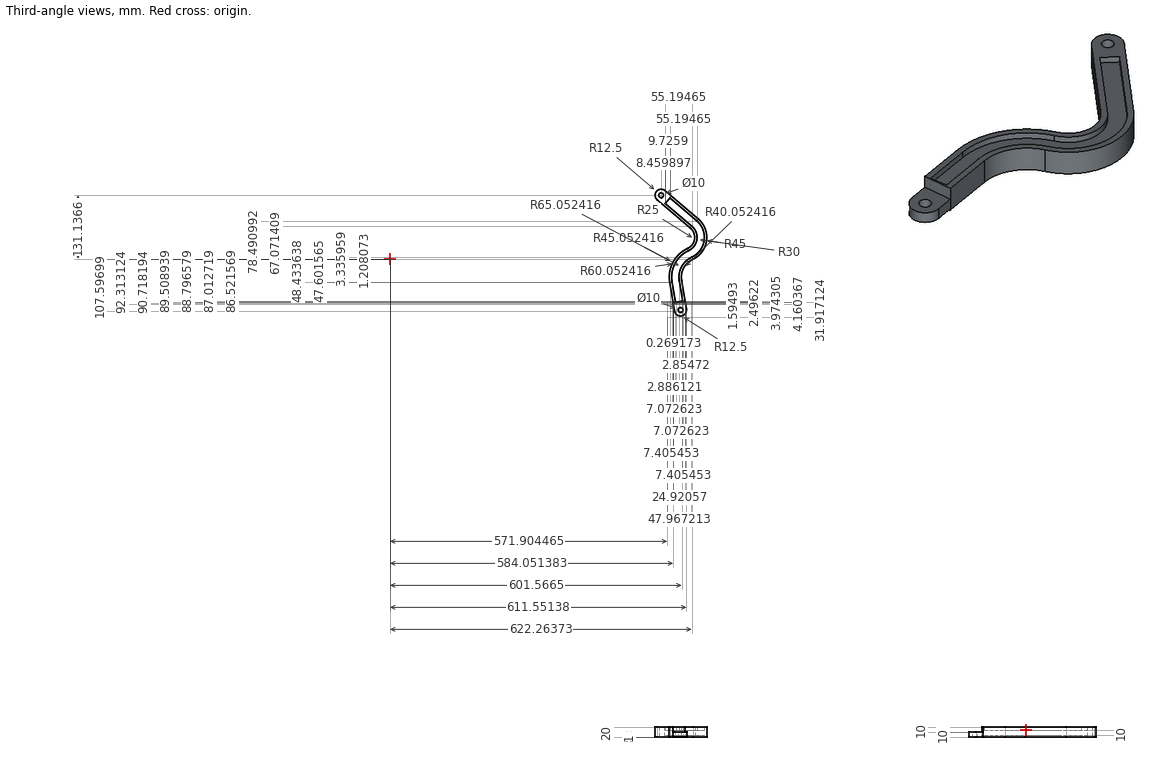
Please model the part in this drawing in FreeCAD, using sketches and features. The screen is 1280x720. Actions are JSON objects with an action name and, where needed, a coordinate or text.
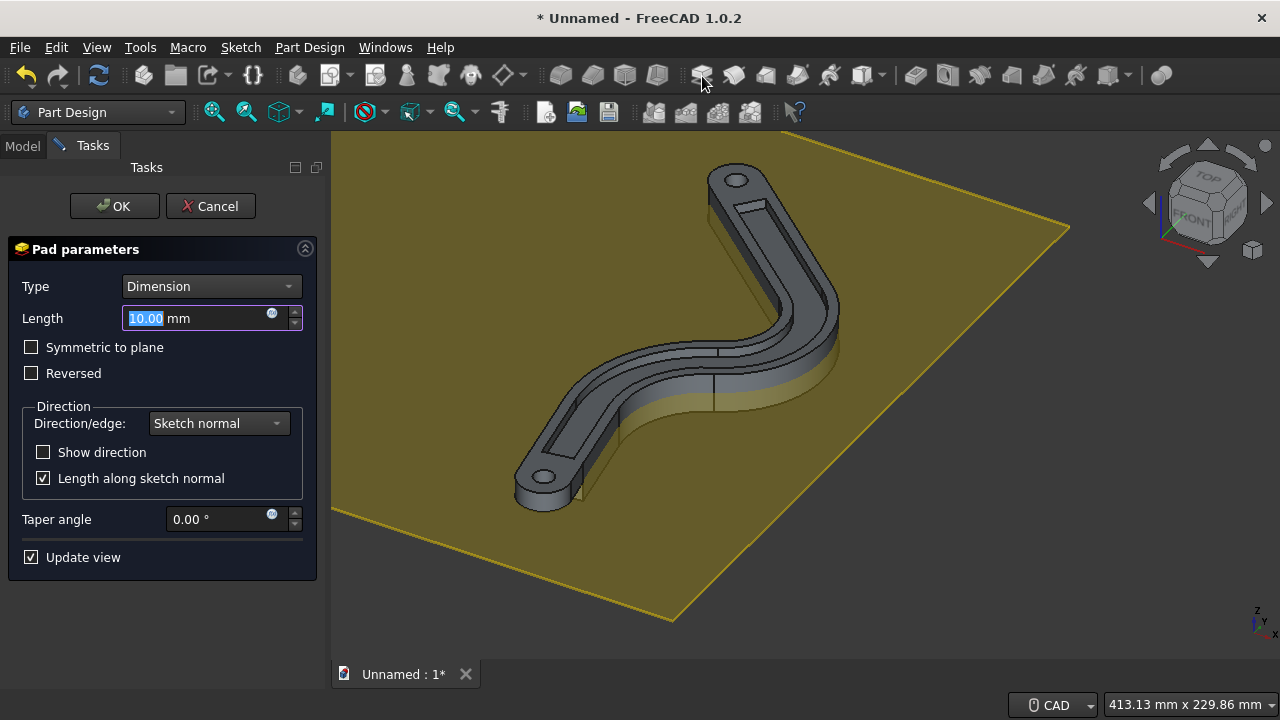
{"action": "type", "text": "10"}
{"action": "key", "text": "Tab"}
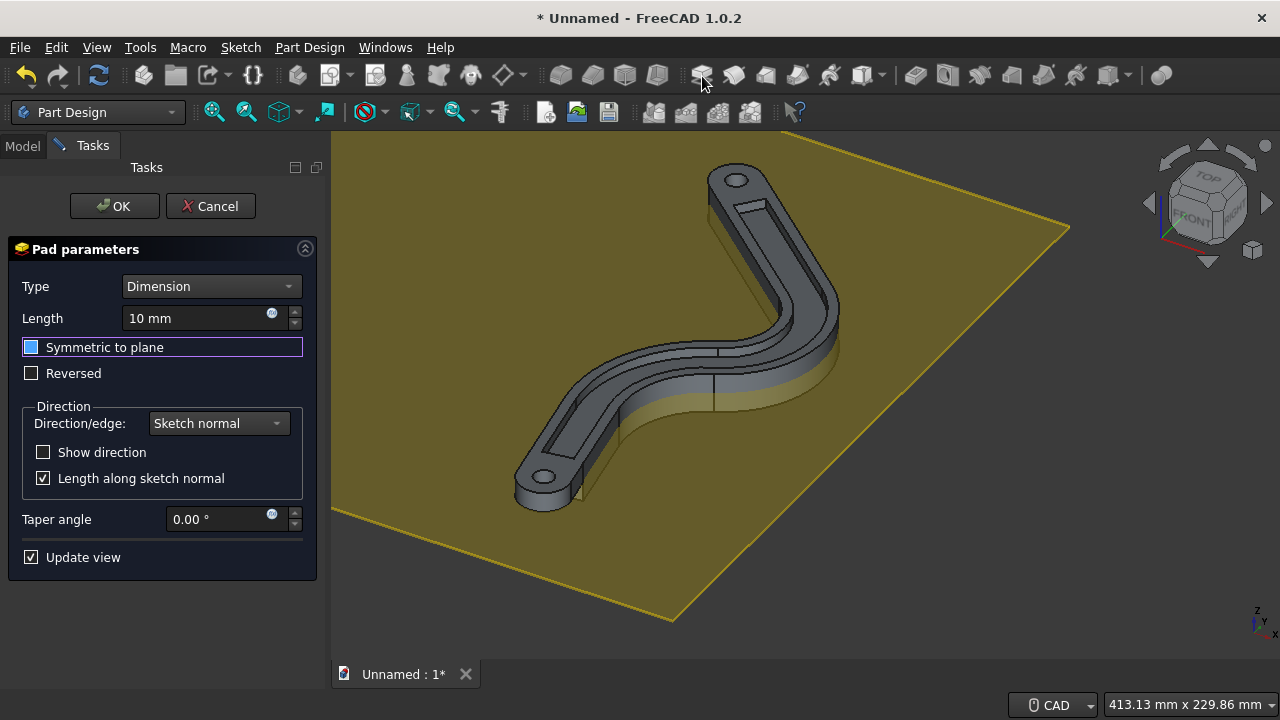
{"action": "left_click", "coordinate": [30, 373]}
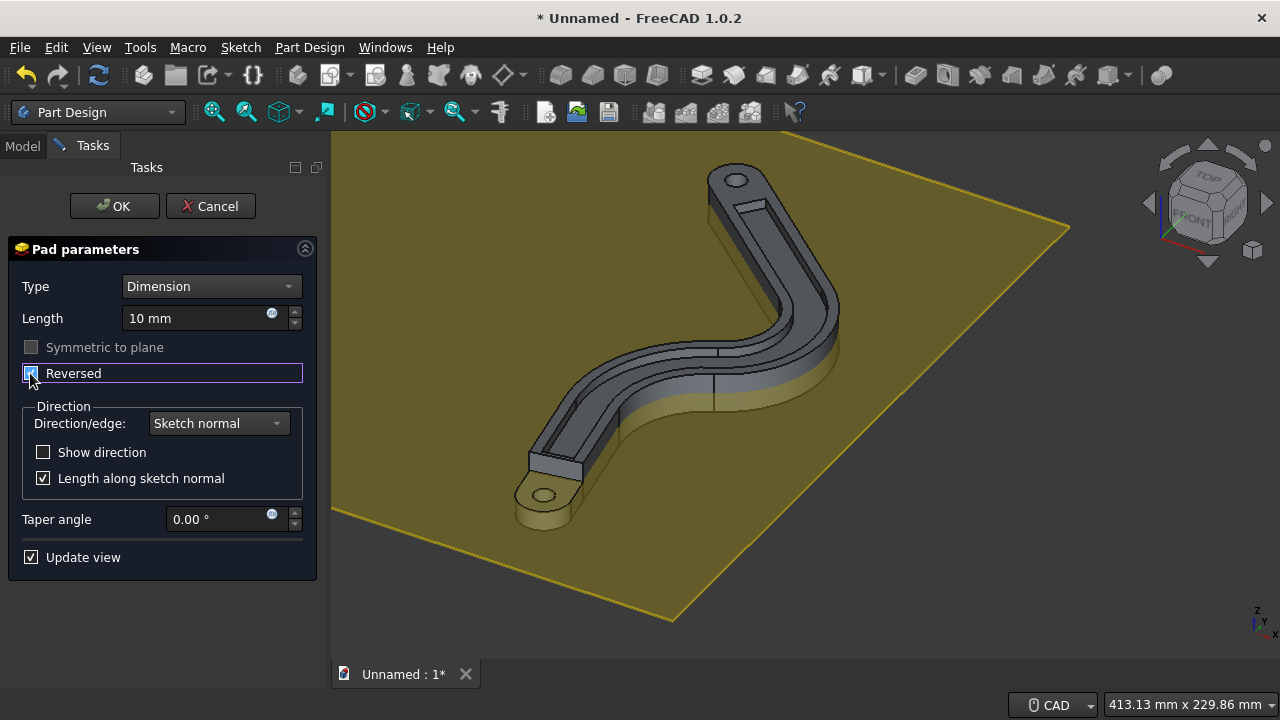
{"action": "left_click", "coordinate": [115, 206]}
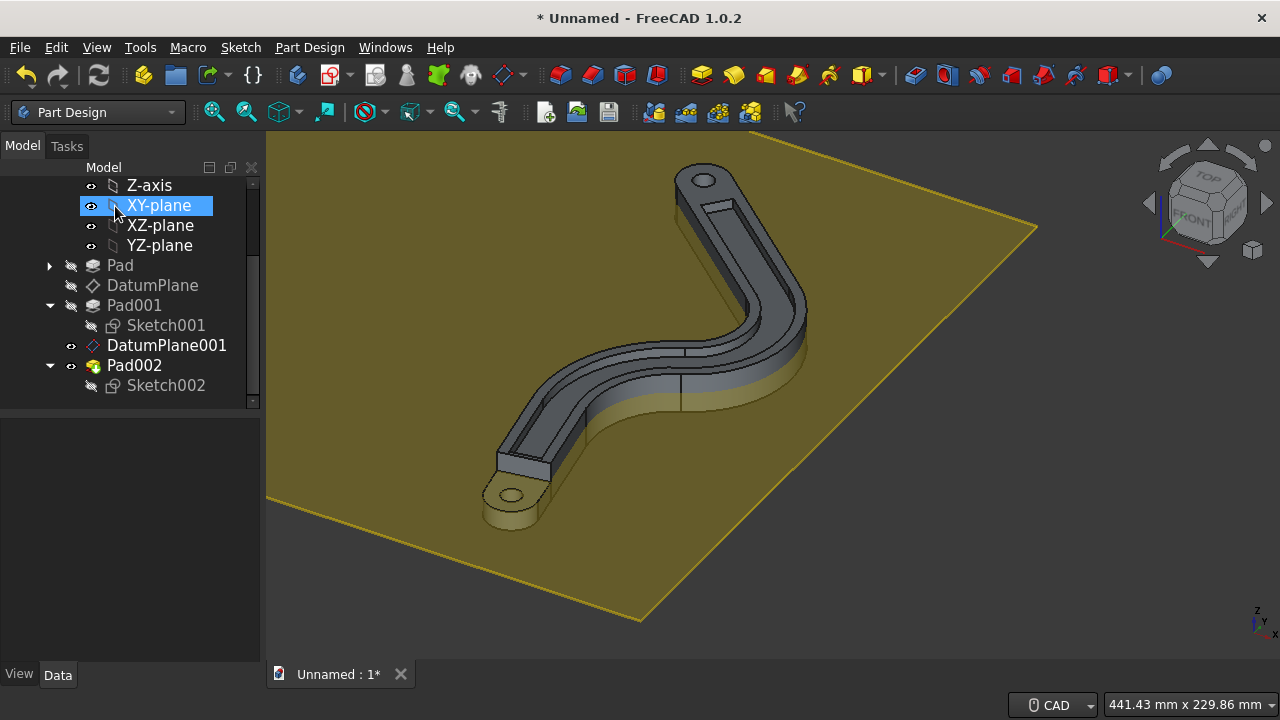
{"action": "left_click", "coordinate": [116, 346]}
{"action": "key", "text": "space"}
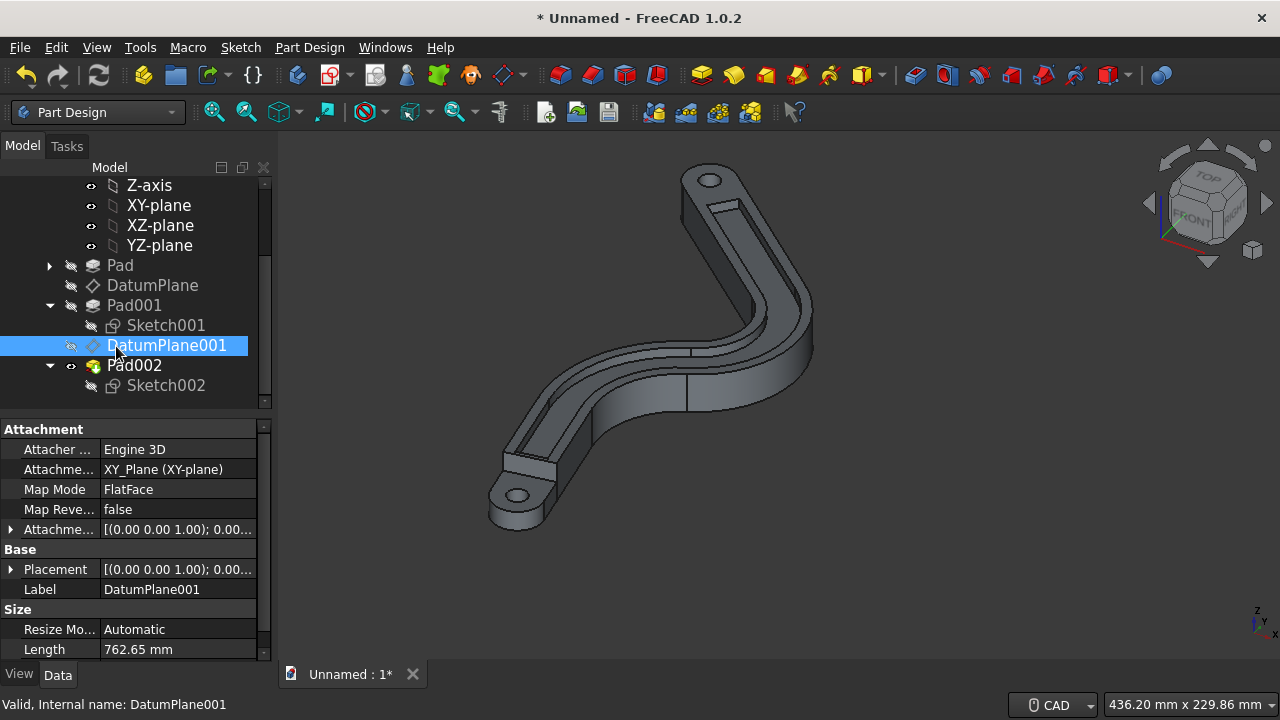
{"action": "key", "text": "5"}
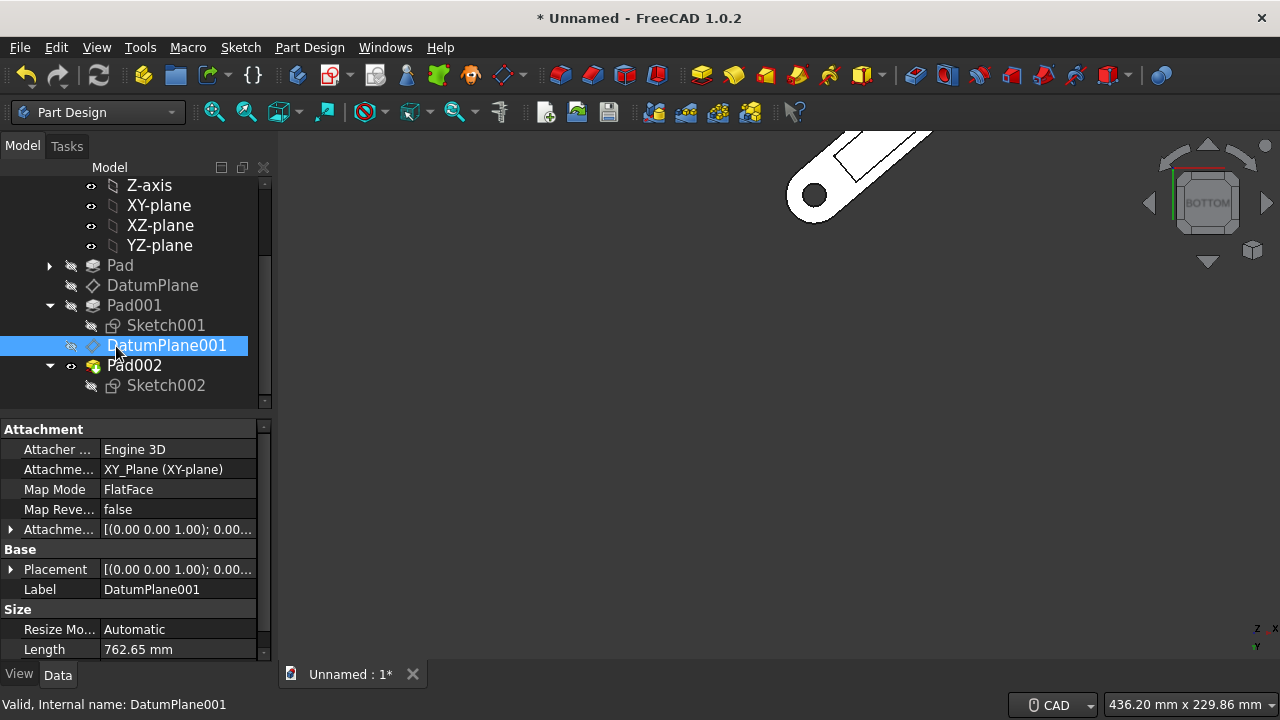
{"action": "left_click", "coordinate": [216, 112]}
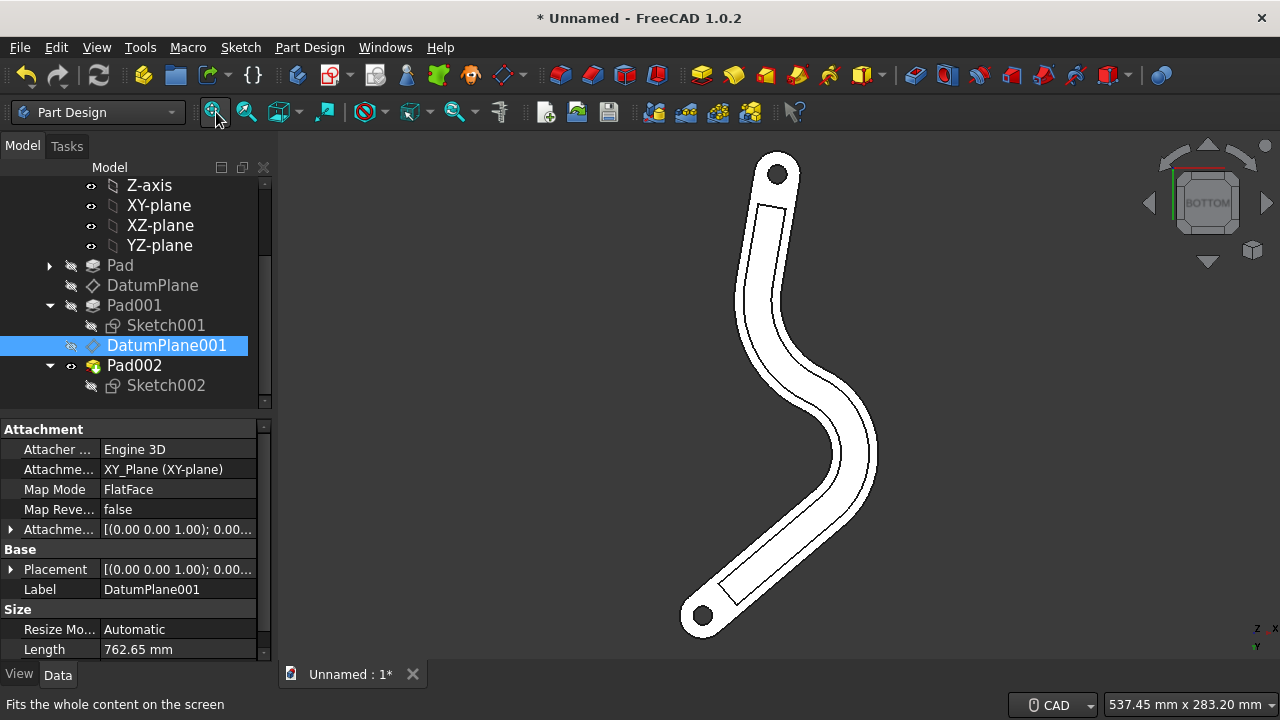
{"action": "left_click", "coordinate": [722, 603]}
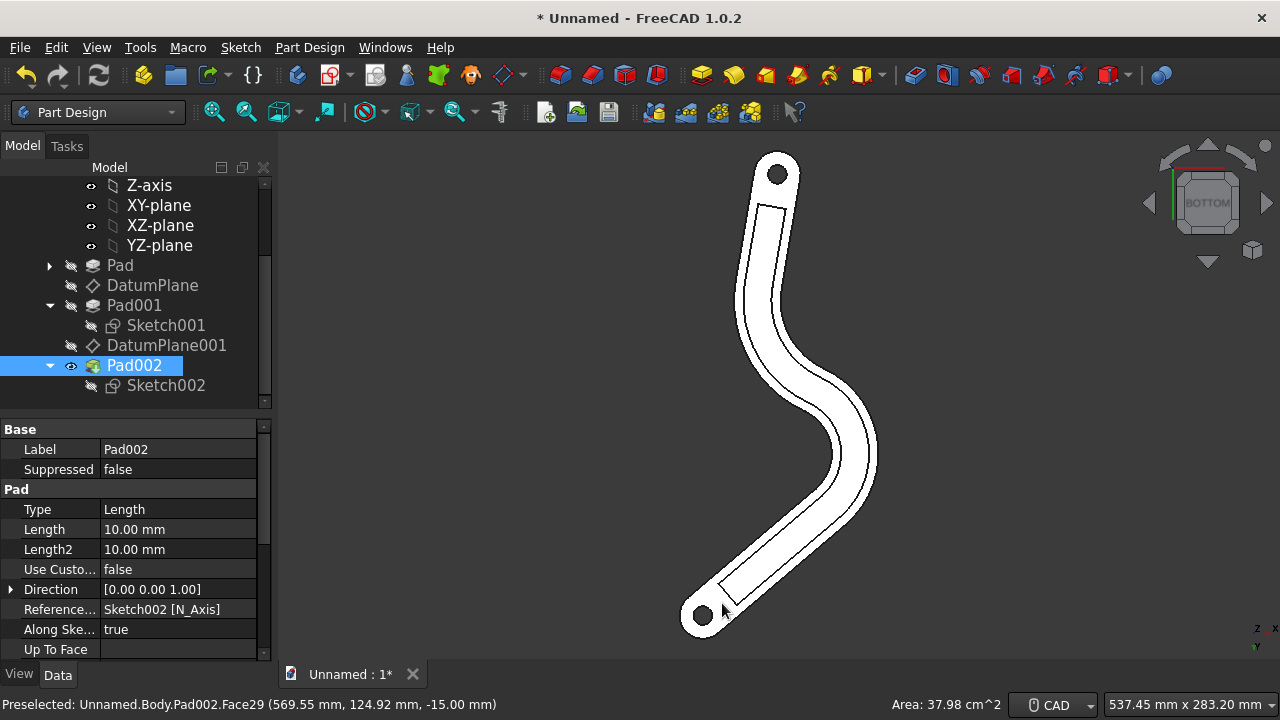
{"action": "left_click", "coordinate": [330, 76]}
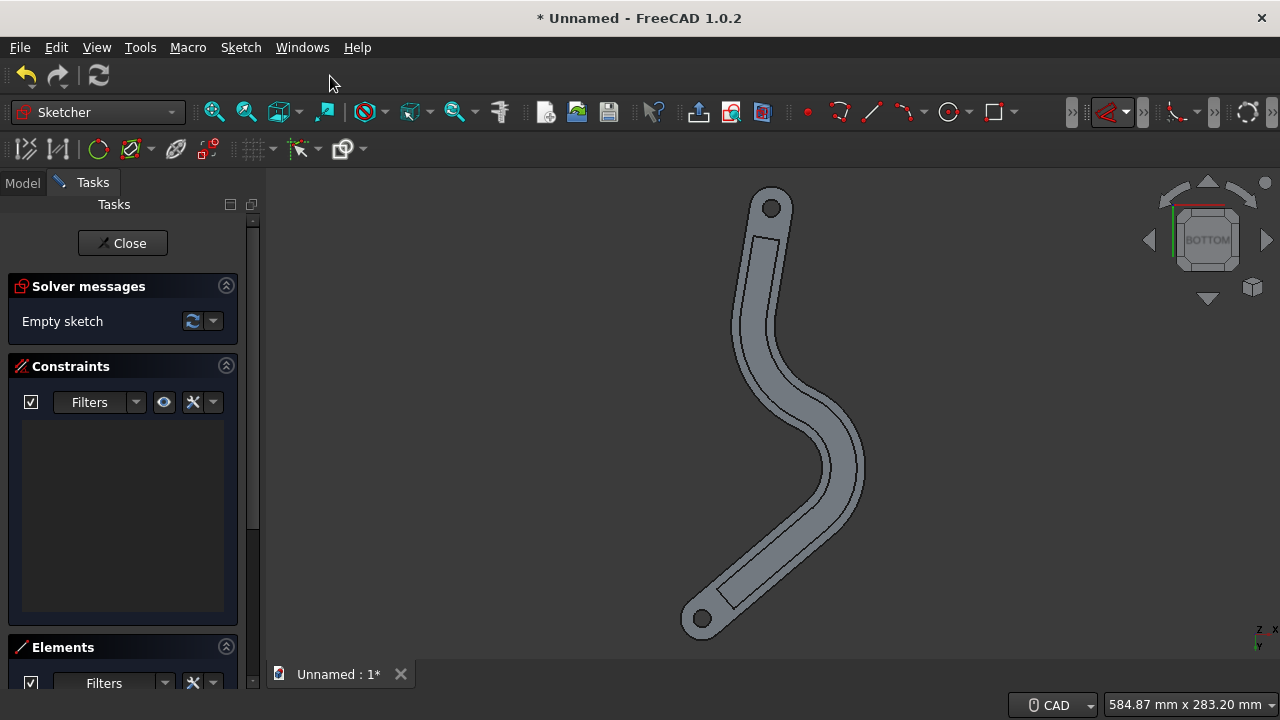
{"action": "scroll", "coordinate": [704, 414], "scroll_direction": "down", "scroll_amount": 5}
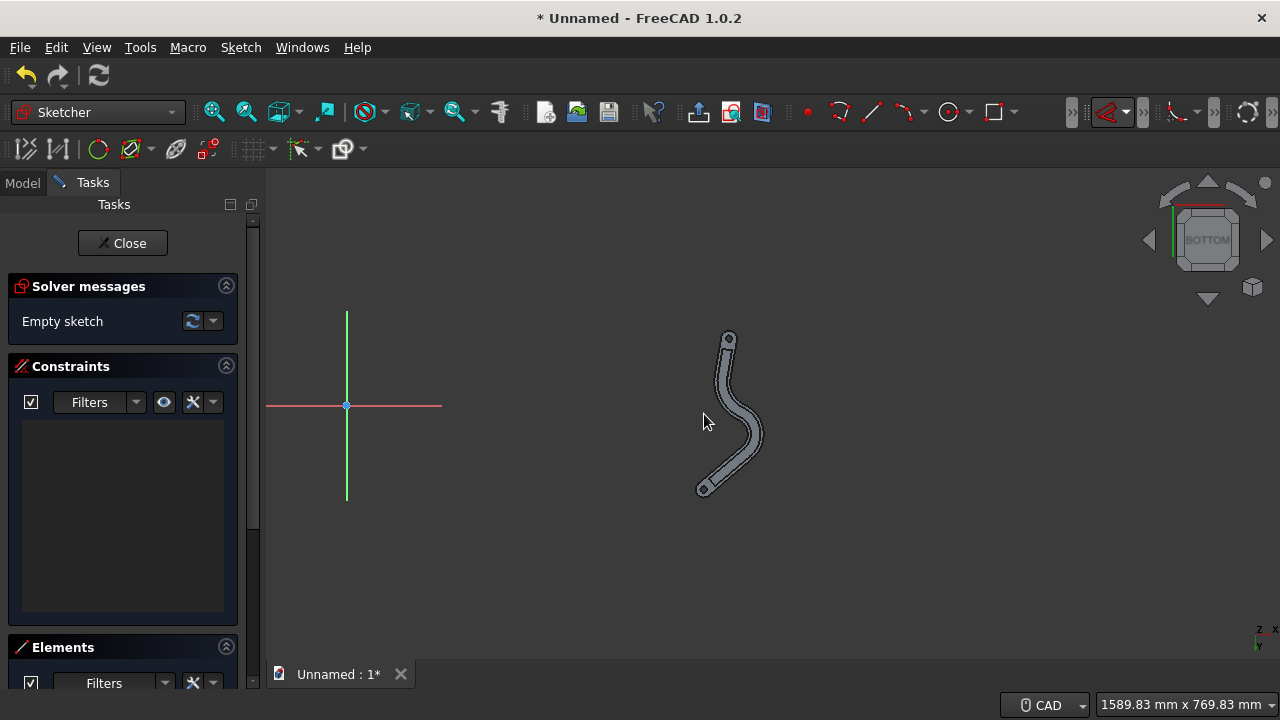
{"action": "scroll", "coordinate": [728, 334], "scroll_direction": "up", "scroll_amount": 14}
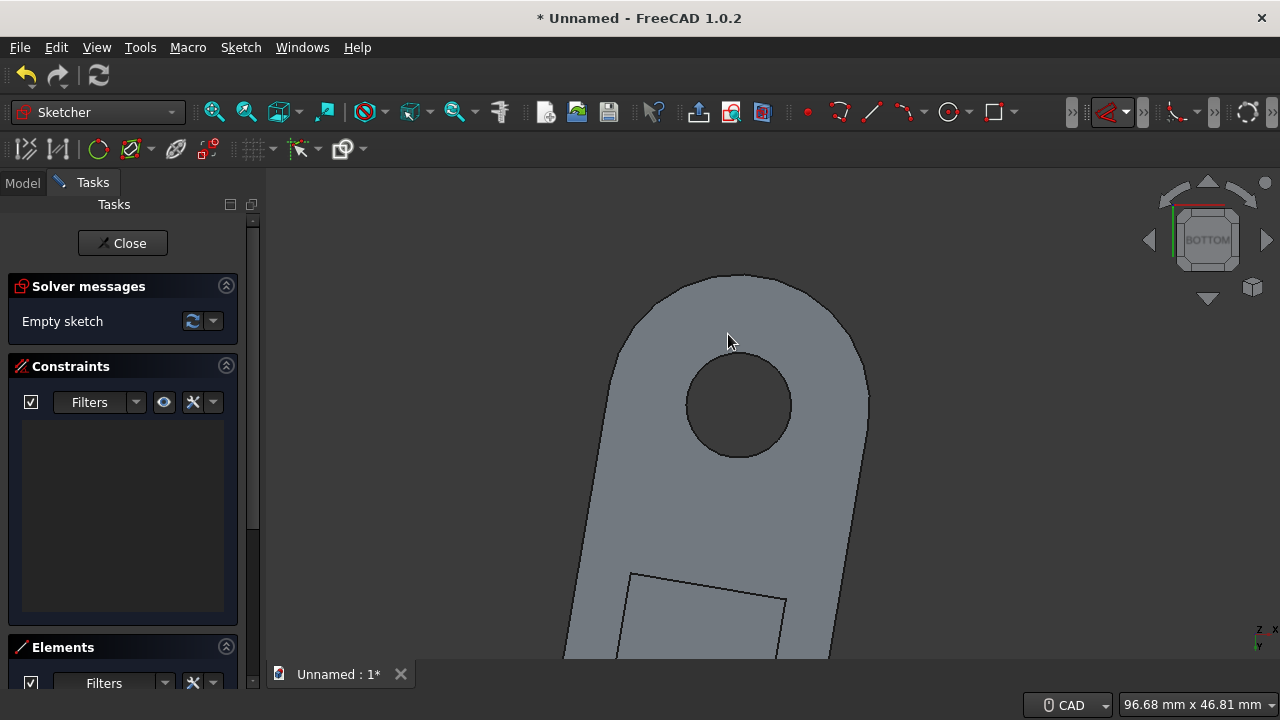
{"action": "left_click", "coordinate": [994, 112]}